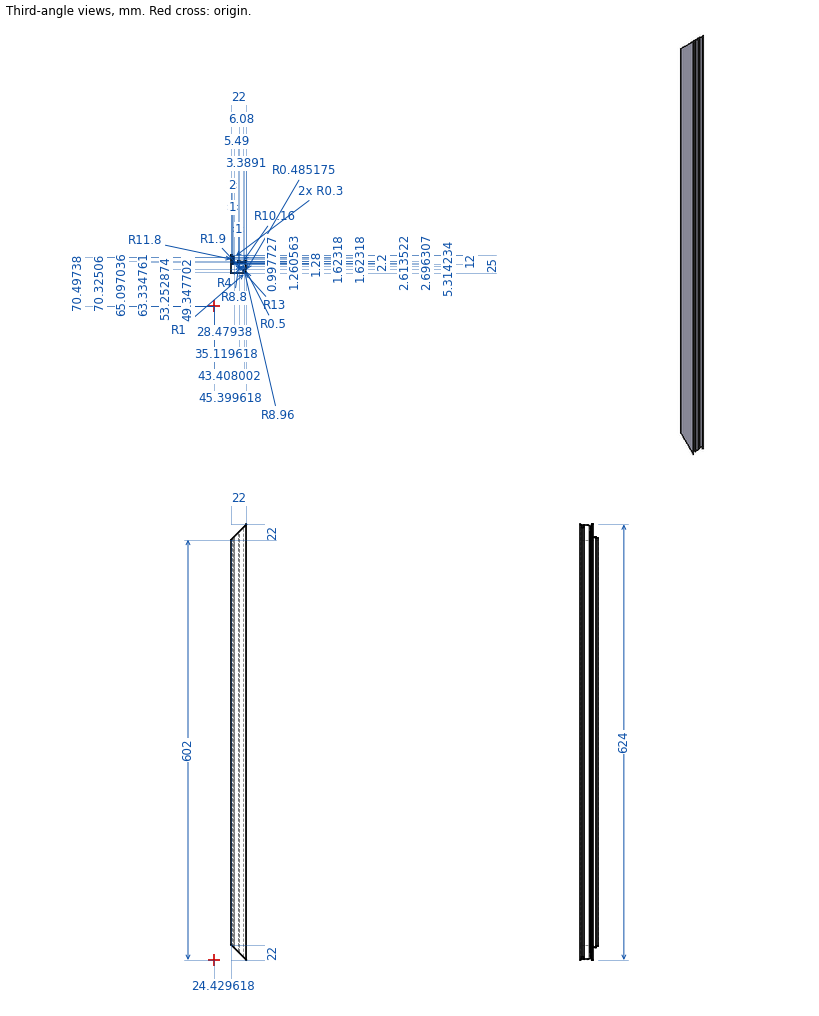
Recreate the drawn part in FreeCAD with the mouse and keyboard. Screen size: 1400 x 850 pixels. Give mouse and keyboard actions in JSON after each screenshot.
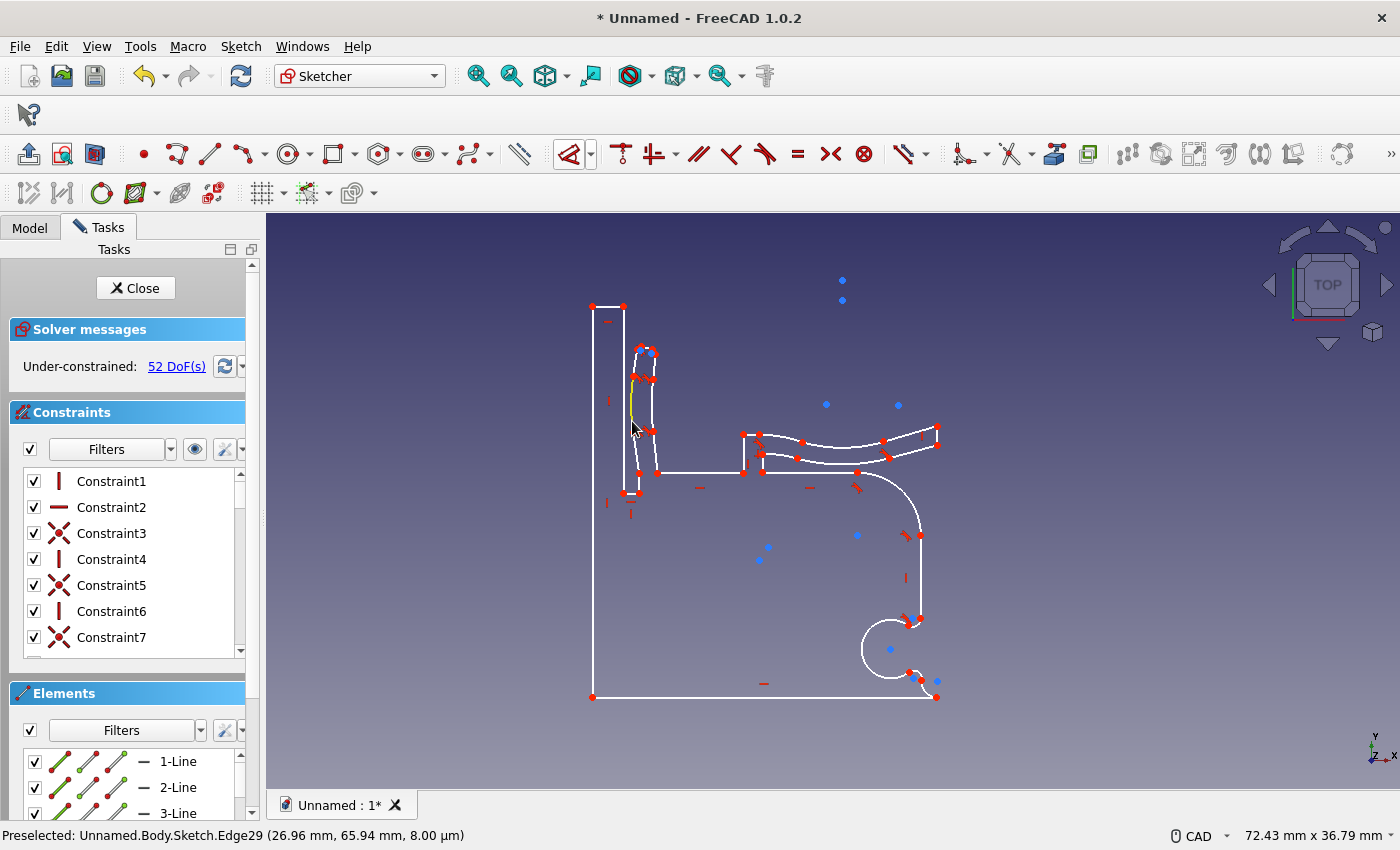
{"action": "left_click", "coordinate": [696, 698]}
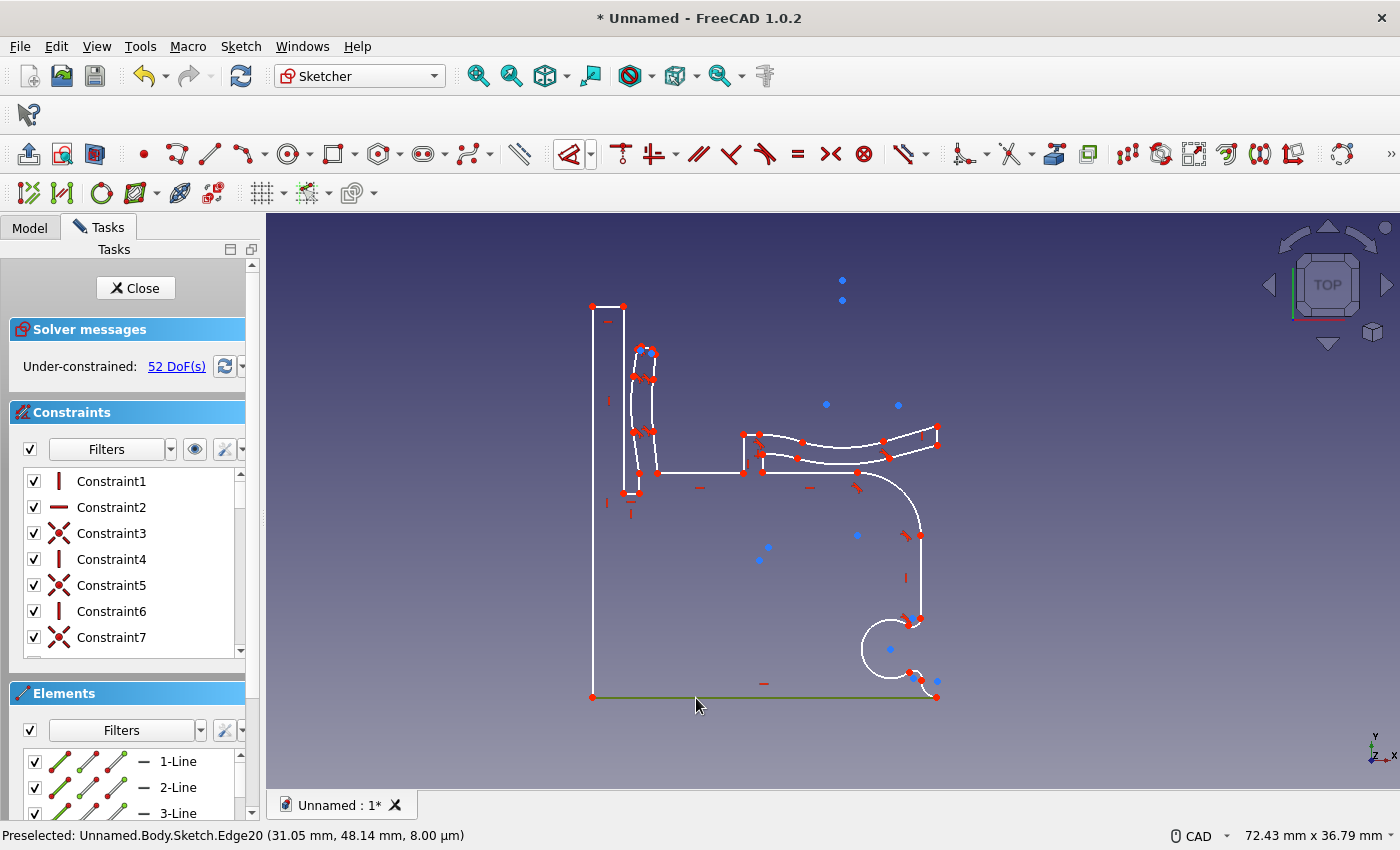
{"action": "scroll", "coordinate": [923, 688], "scroll_direction": "up", "scroll_amount": 3}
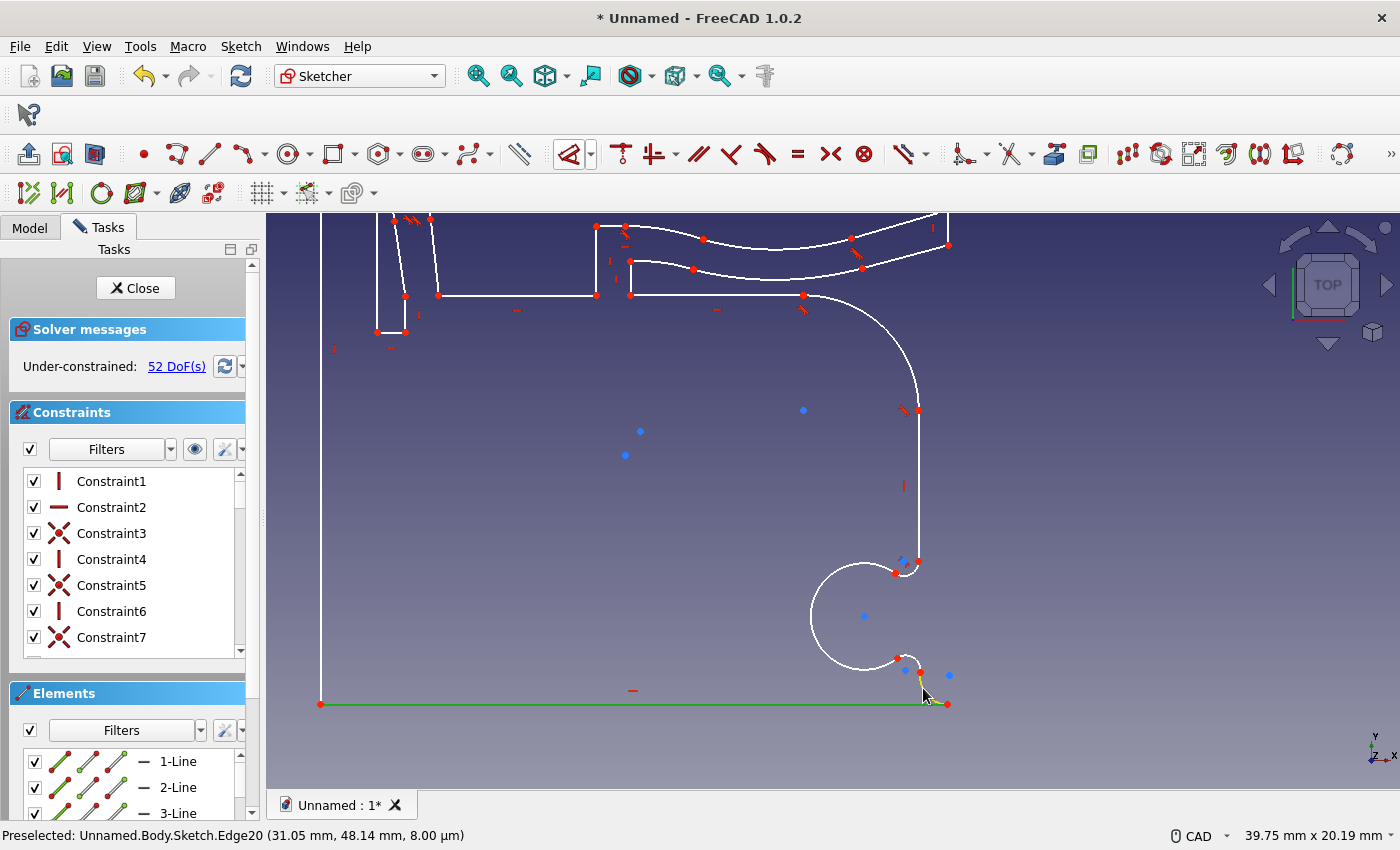
{"action": "left_click", "coordinate": [922, 687]}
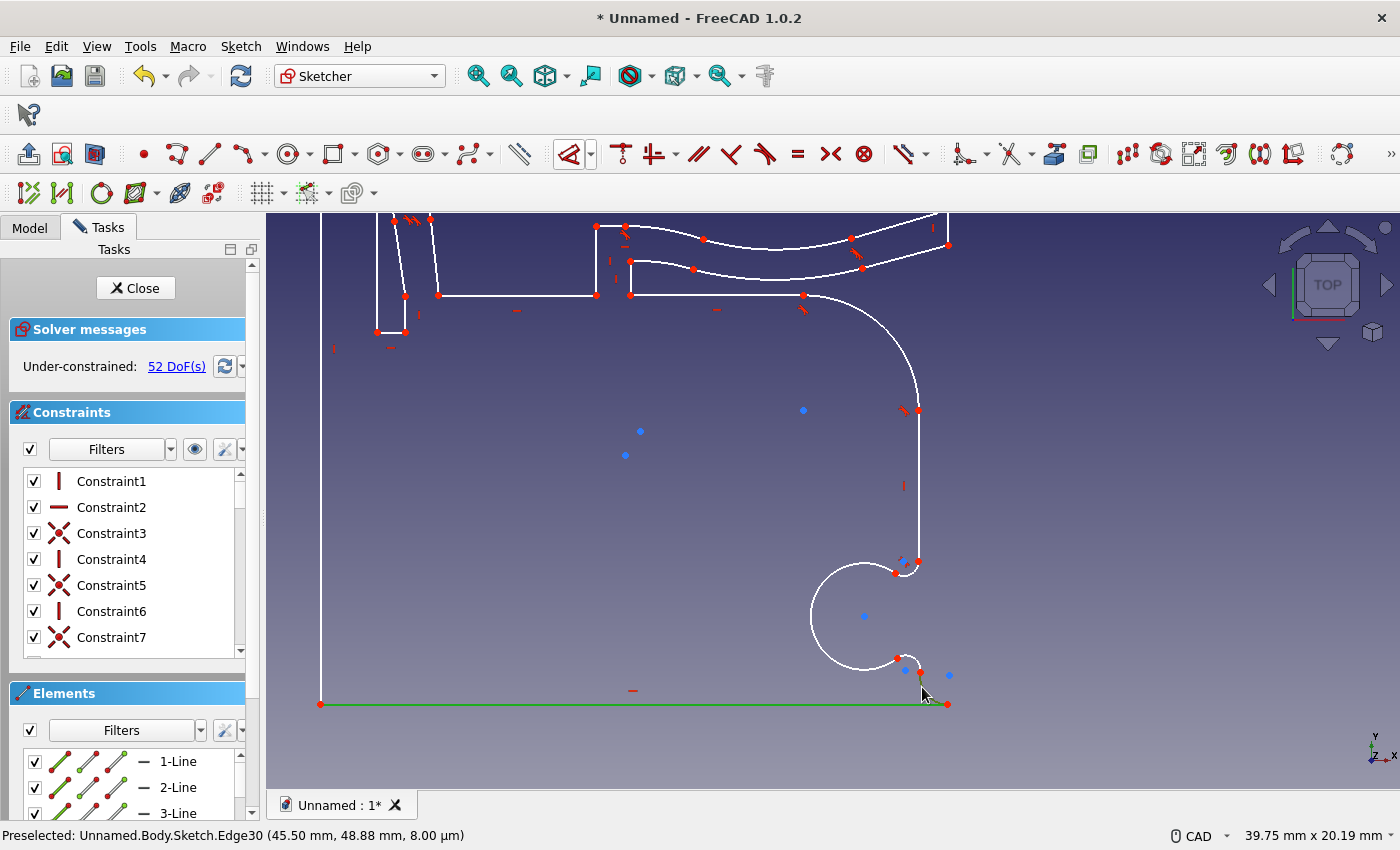
{"action": "key", "text": "t"}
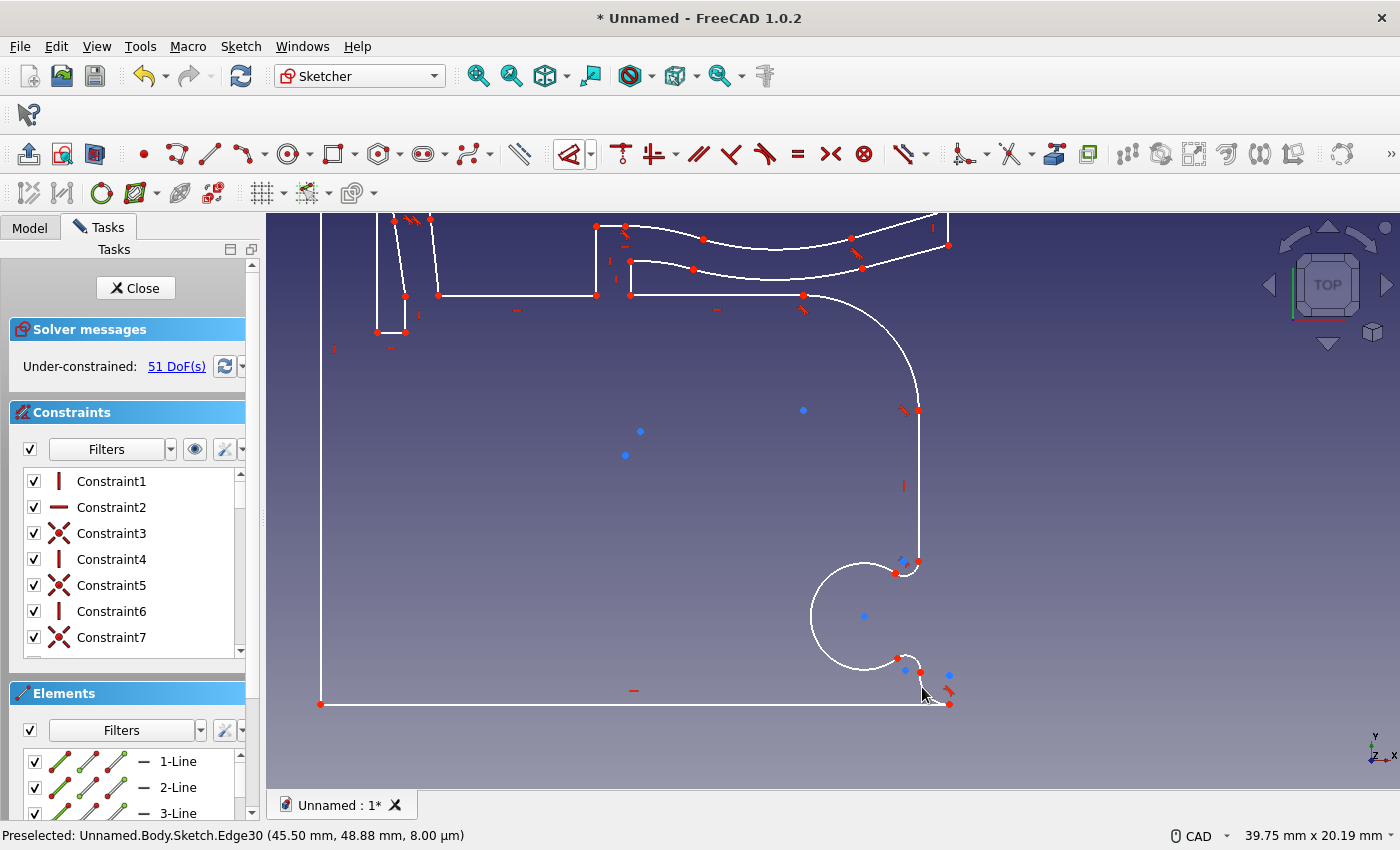
{"action": "left_click", "coordinate": [675, 265]}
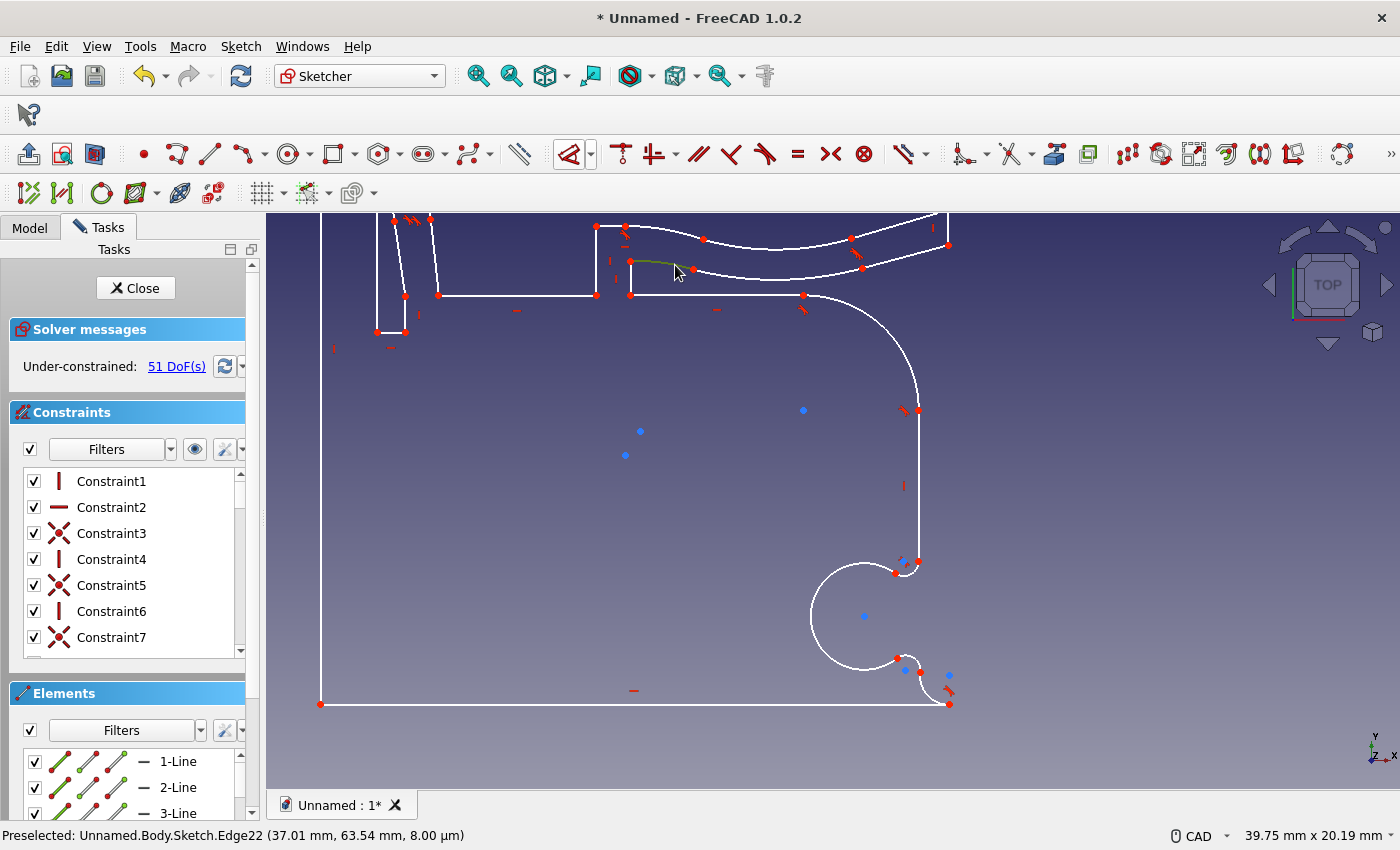
{"action": "left_click", "coordinate": [744, 278]}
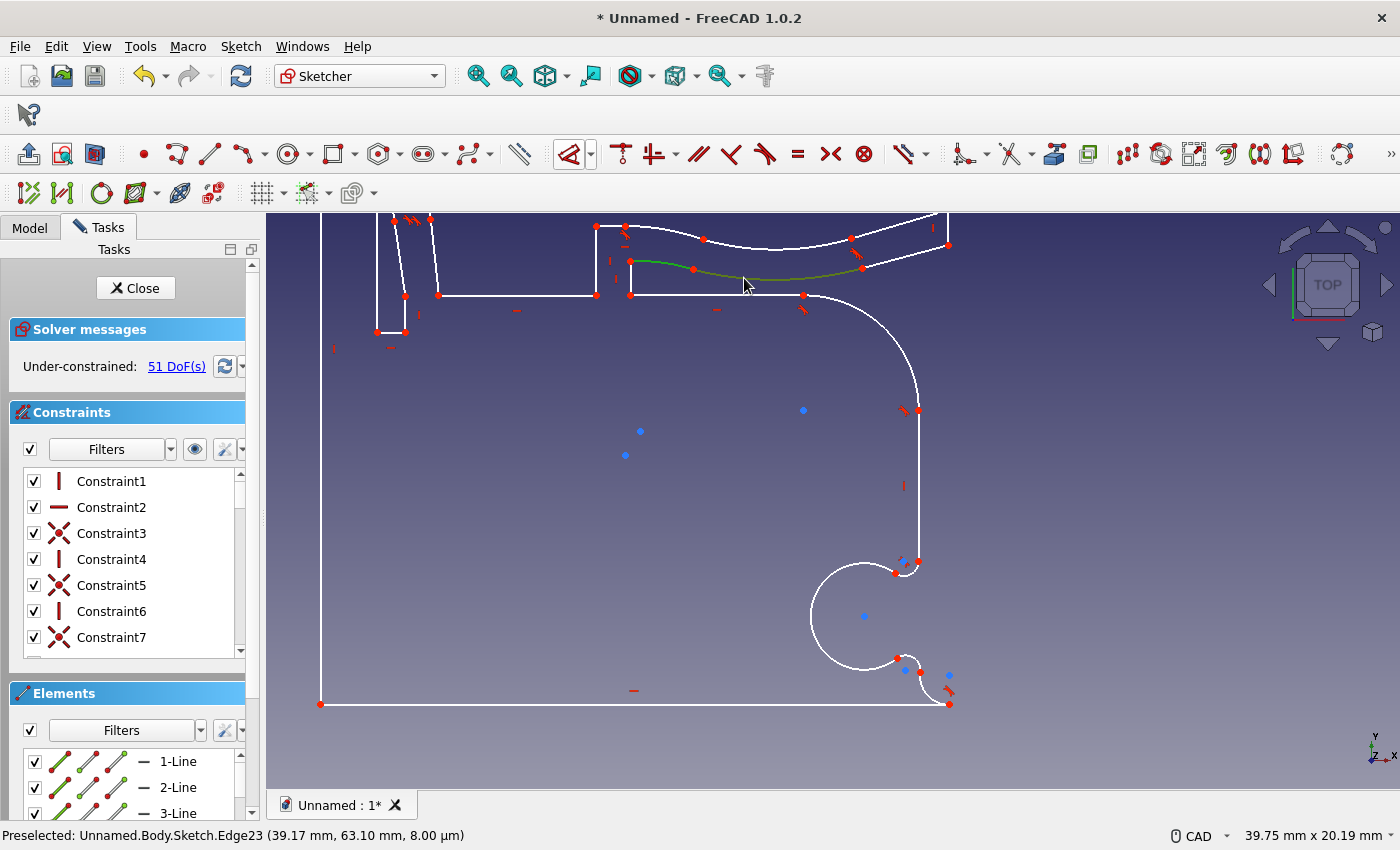
{"action": "key", "text": "t"}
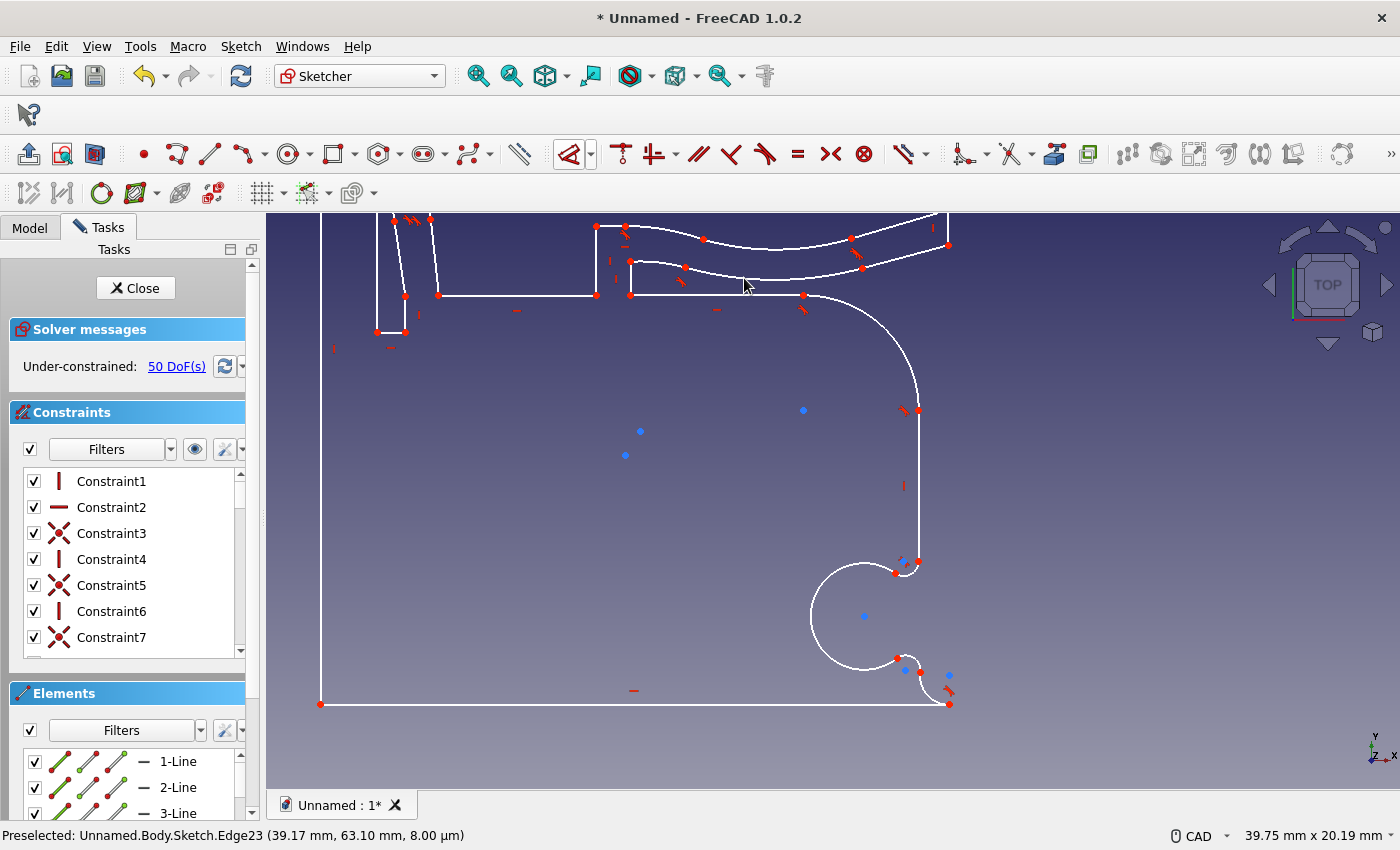
{"action": "left_click", "coordinate": [747, 248]}